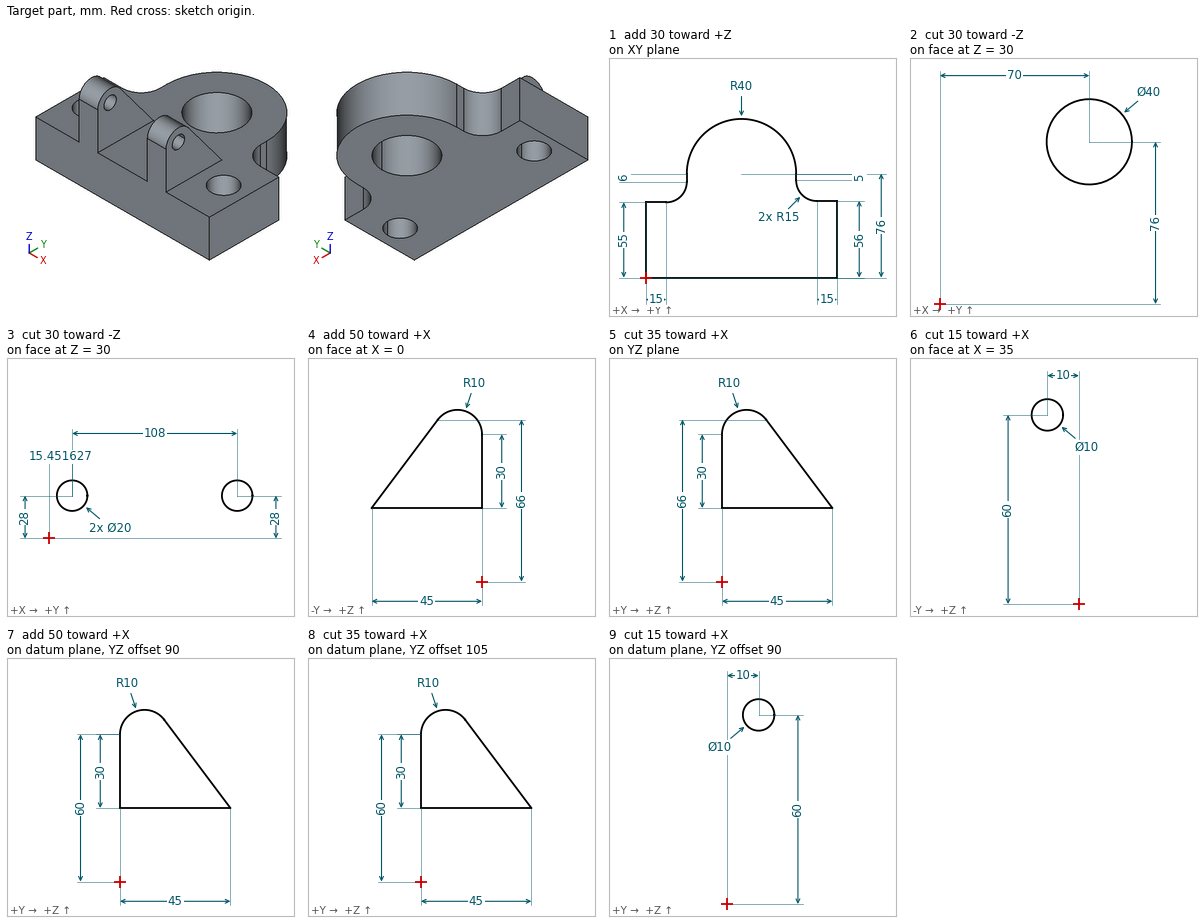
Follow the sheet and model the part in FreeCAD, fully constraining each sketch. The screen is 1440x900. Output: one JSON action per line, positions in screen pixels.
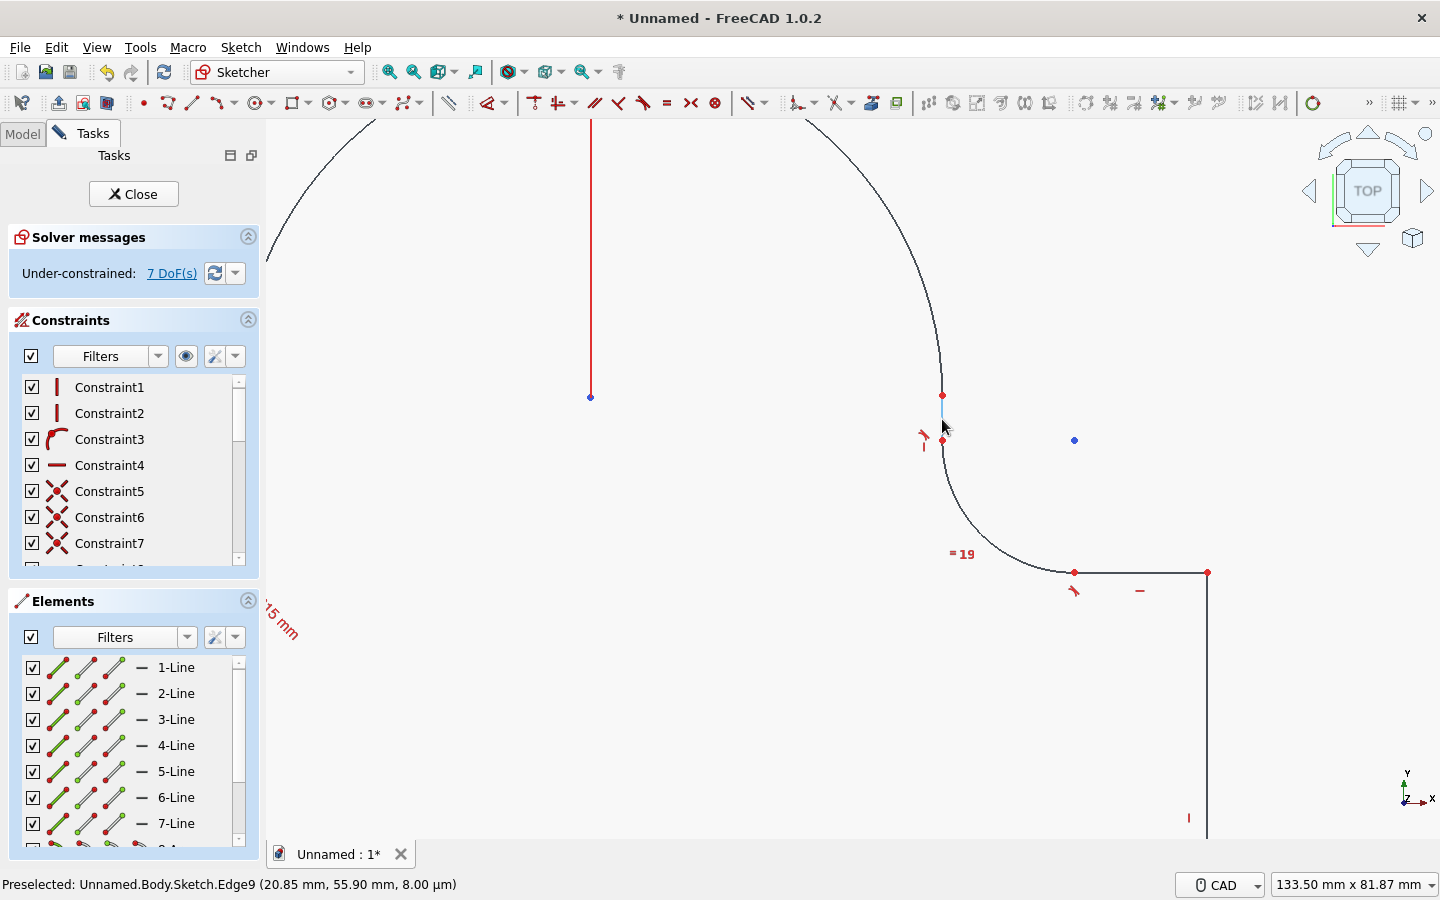
{"action": "left_click", "coordinate": [942, 418]}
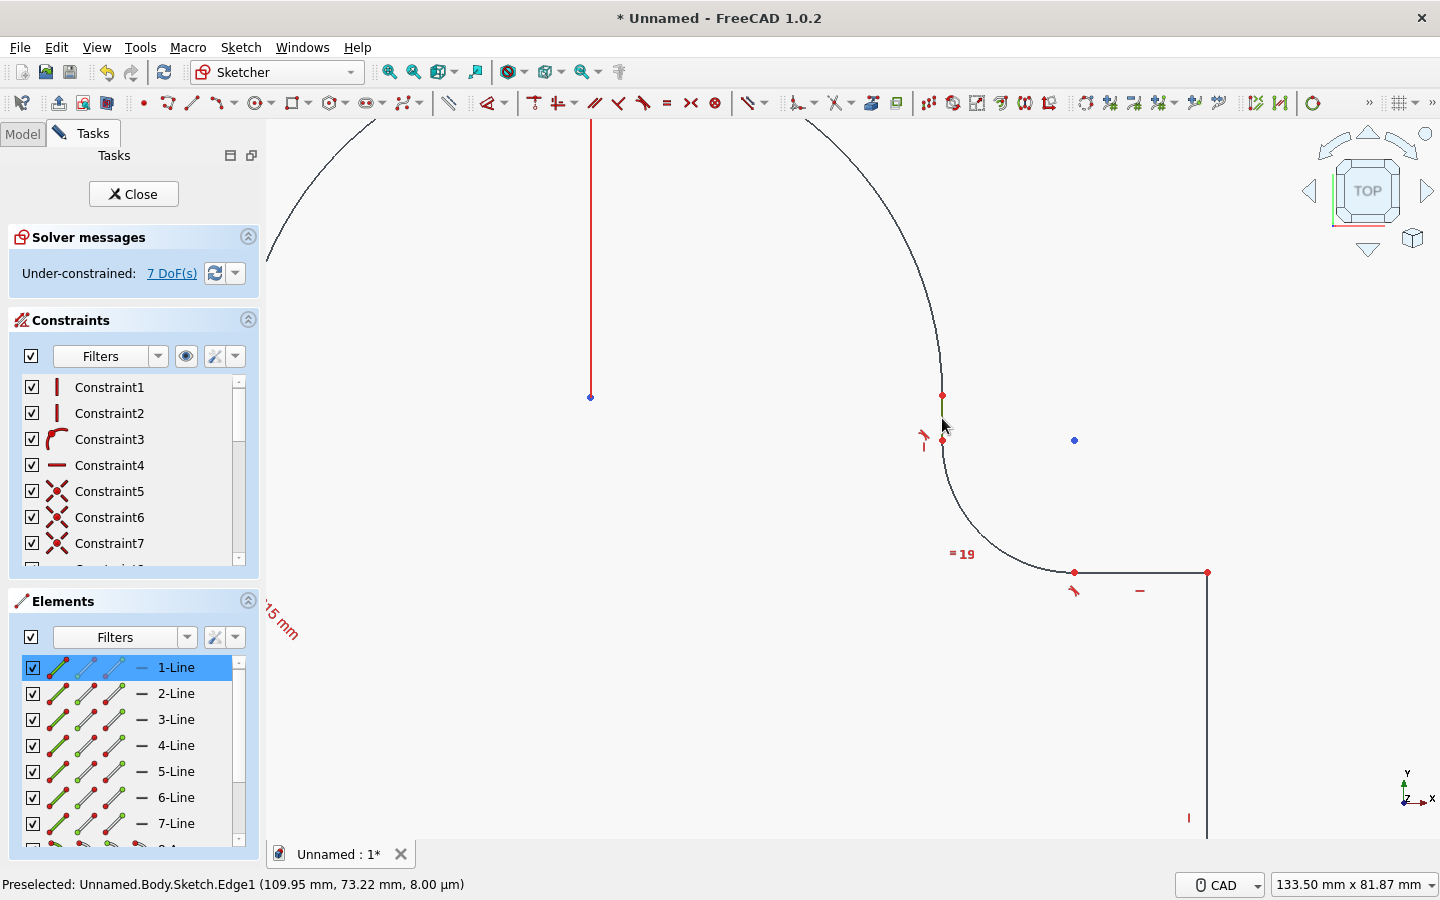
{"action": "key", "text": "i"}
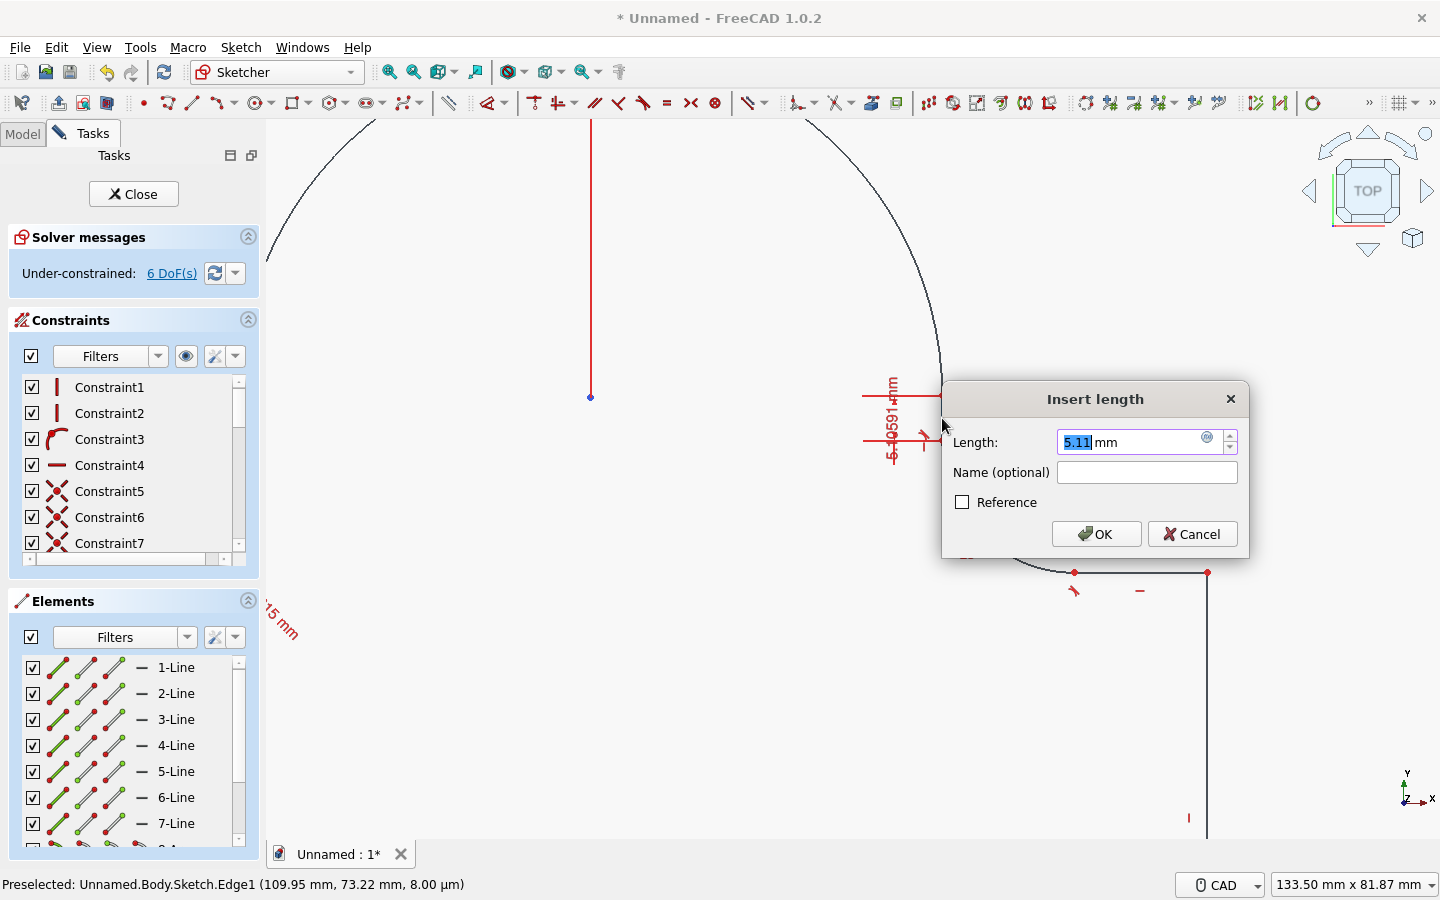
{"action": "type", "text": "5"}
{"action": "key", "text": "Return"}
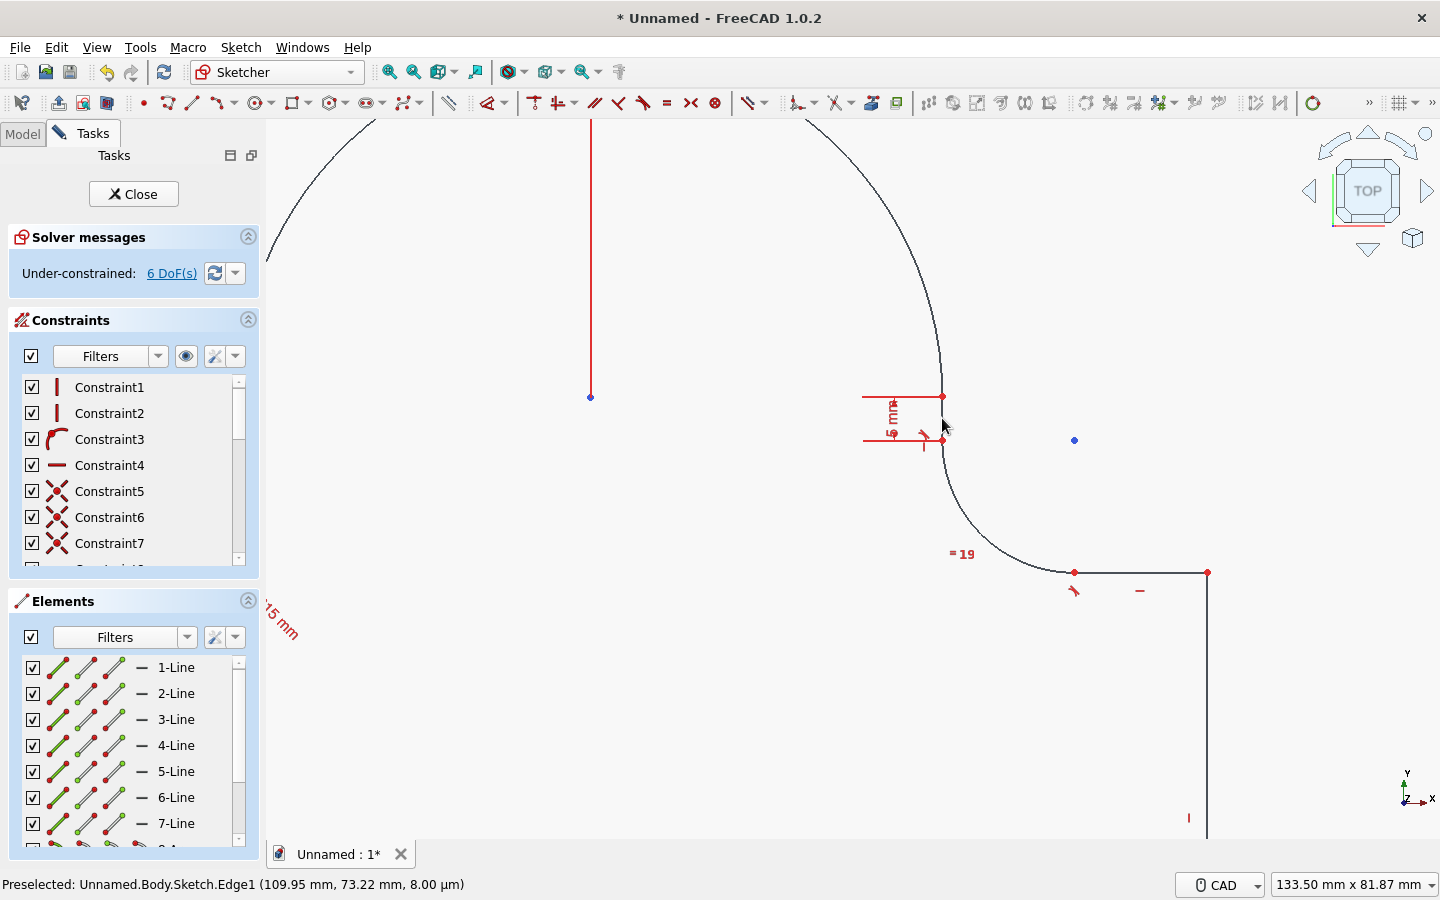
{"action": "scroll", "coordinate": [942, 419], "scroll_direction": "down", "scroll_amount": 4}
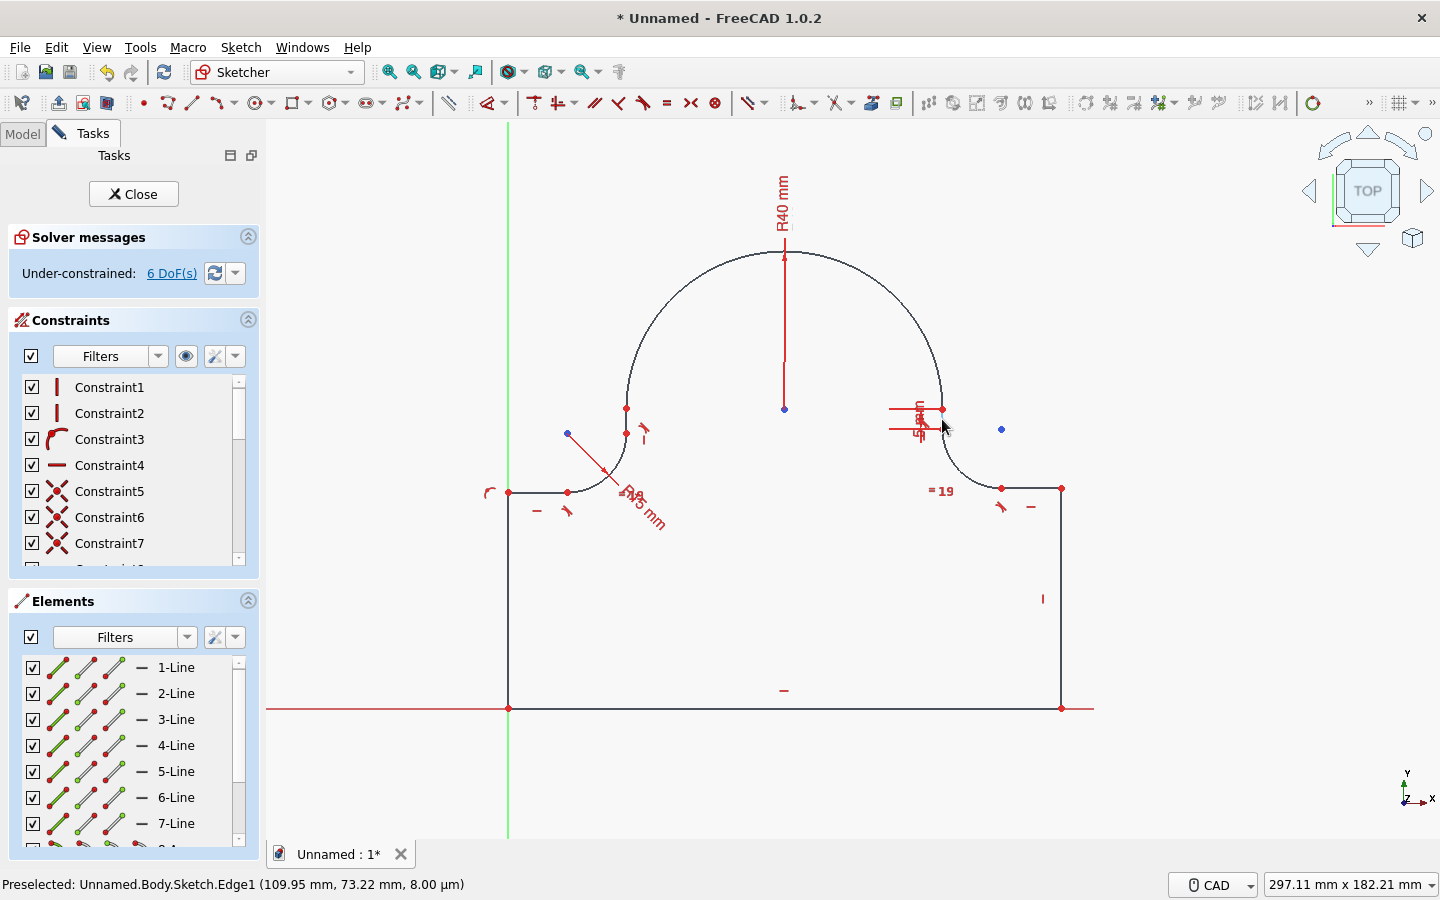
{"action": "scroll", "coordinate": [626, 416], "scroll_direction": "up", "scroll_amount": 4}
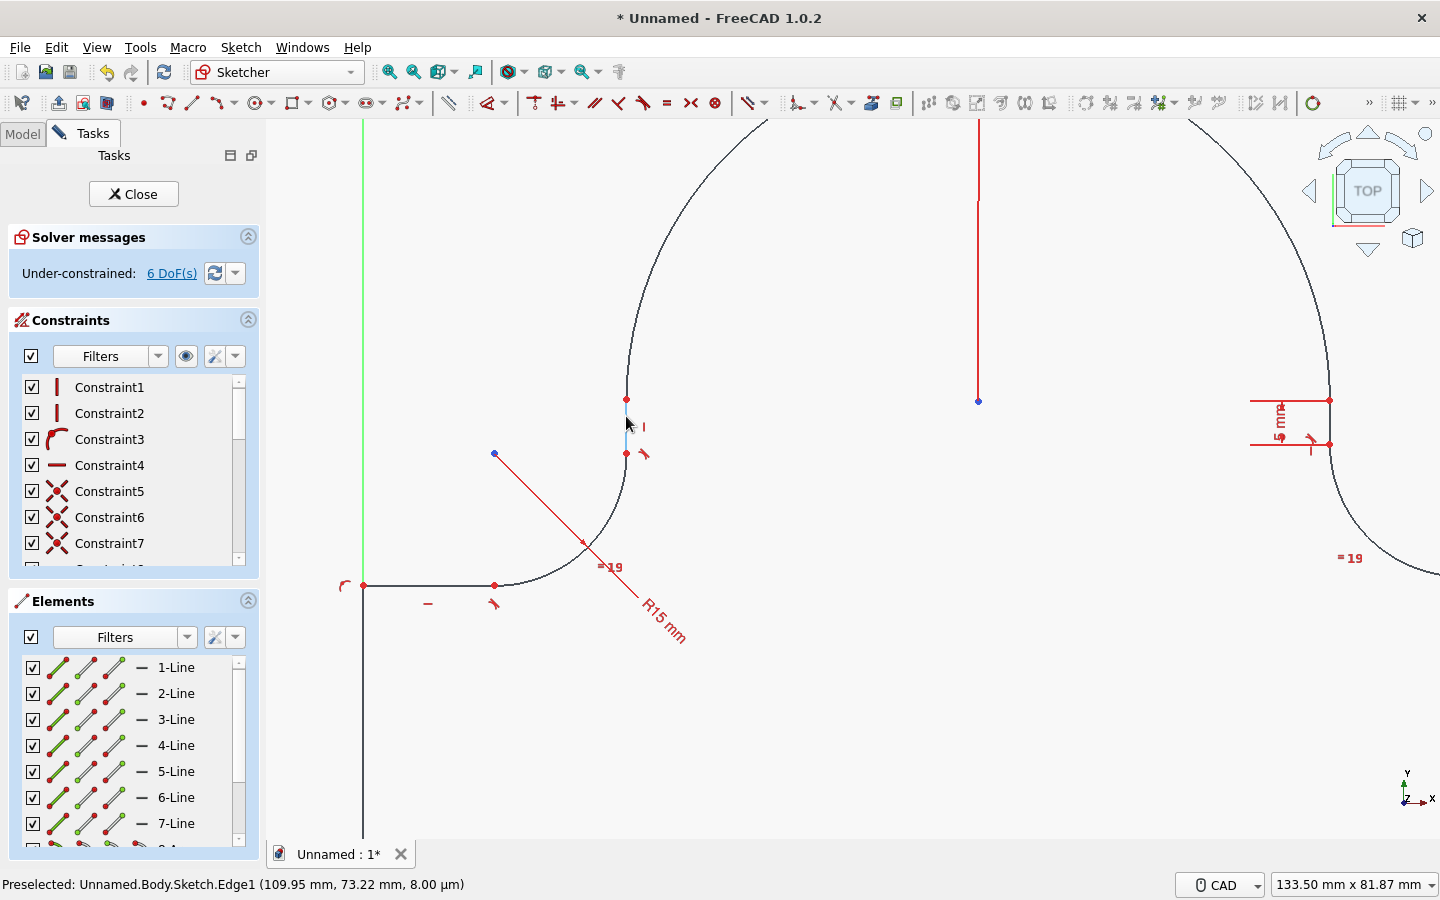
{"action": "left_click", "coordinate": [626, 416]}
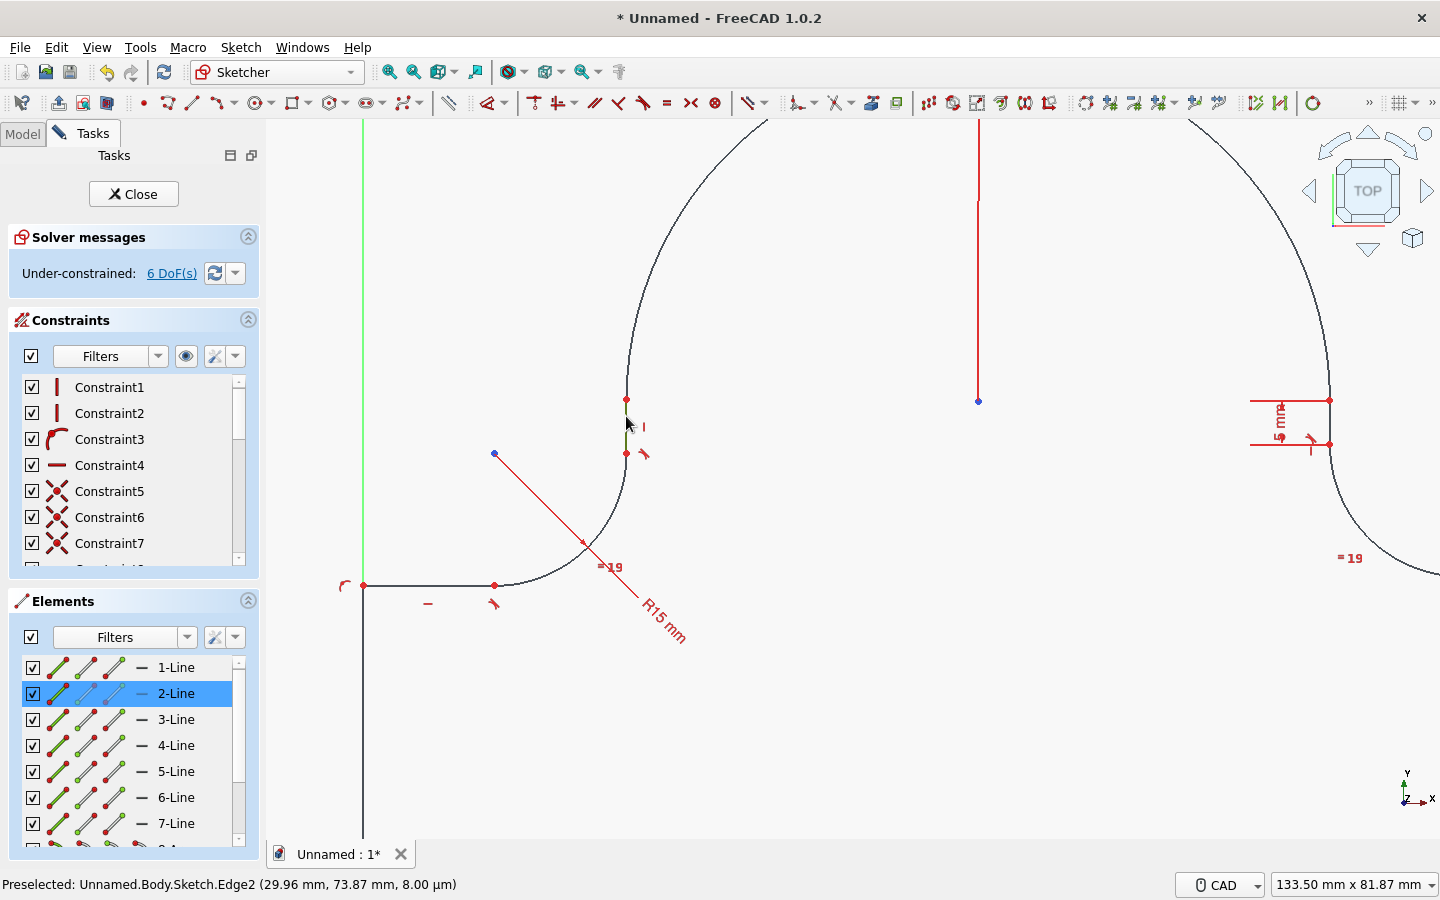
{"action": "key", "text": "i"}